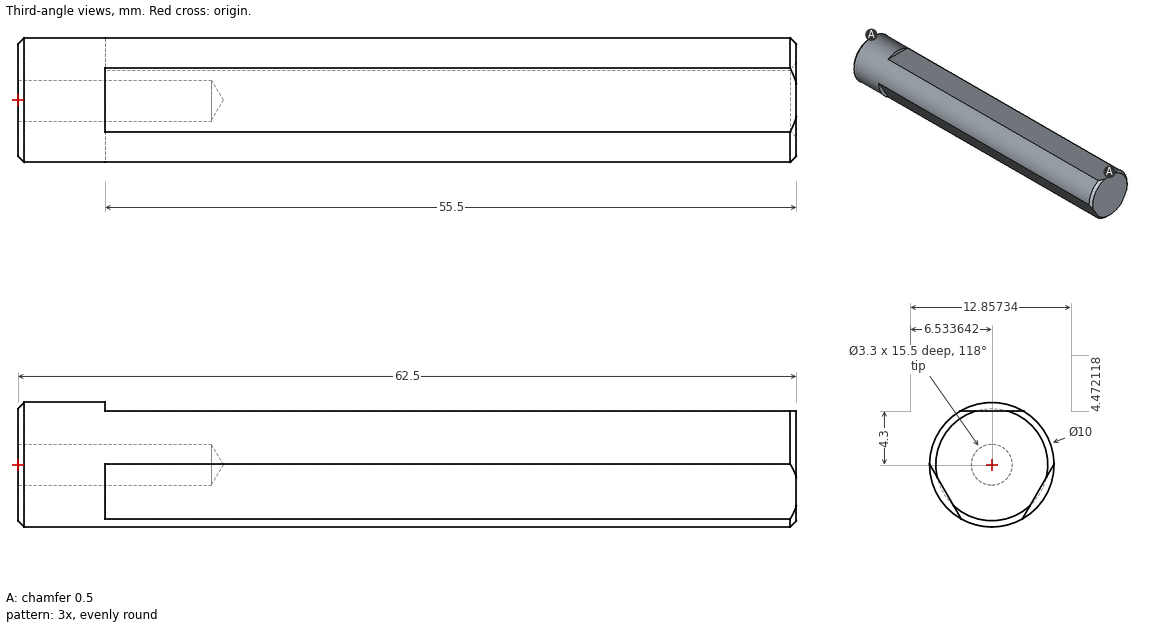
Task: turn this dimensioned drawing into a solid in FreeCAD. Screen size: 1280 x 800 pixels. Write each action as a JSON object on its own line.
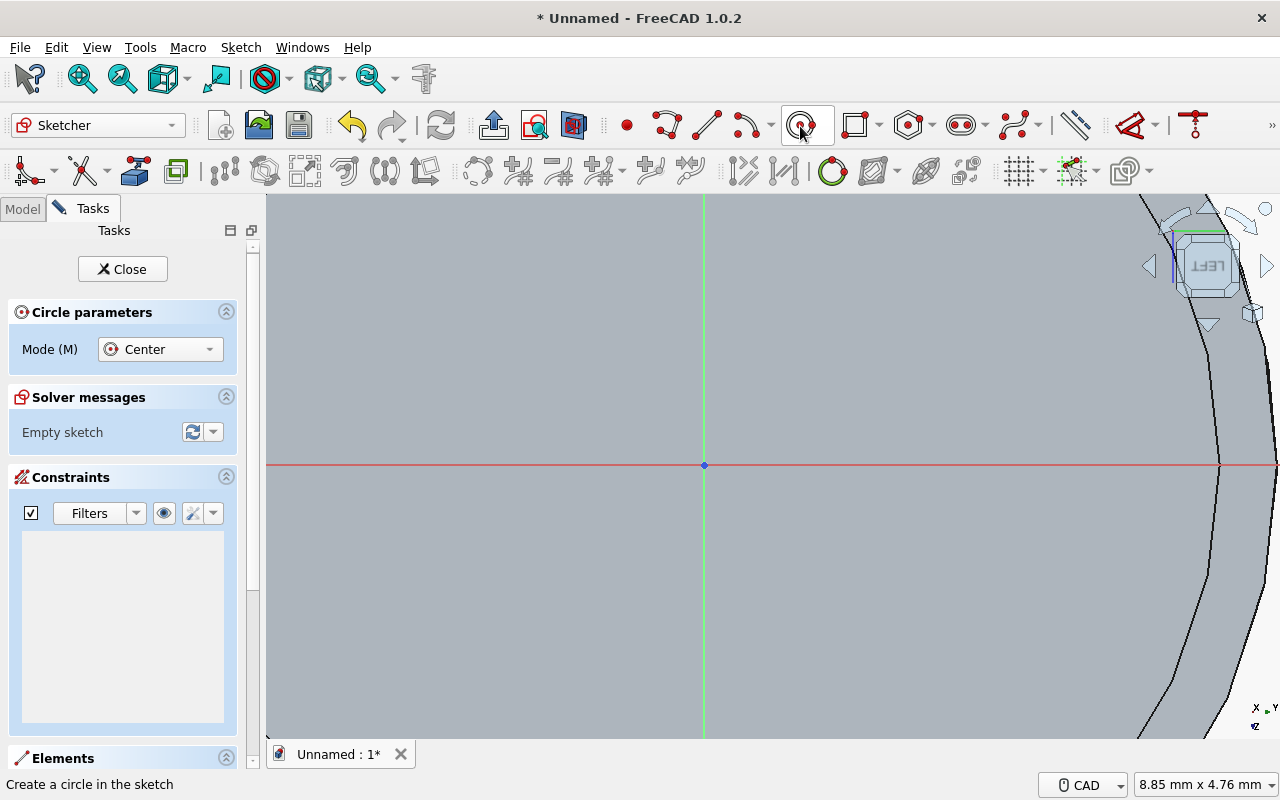
{"action": "left_click", "coordinate": [704, 465]}
{"action": "mouse_move", "coordinate": [838, 331]}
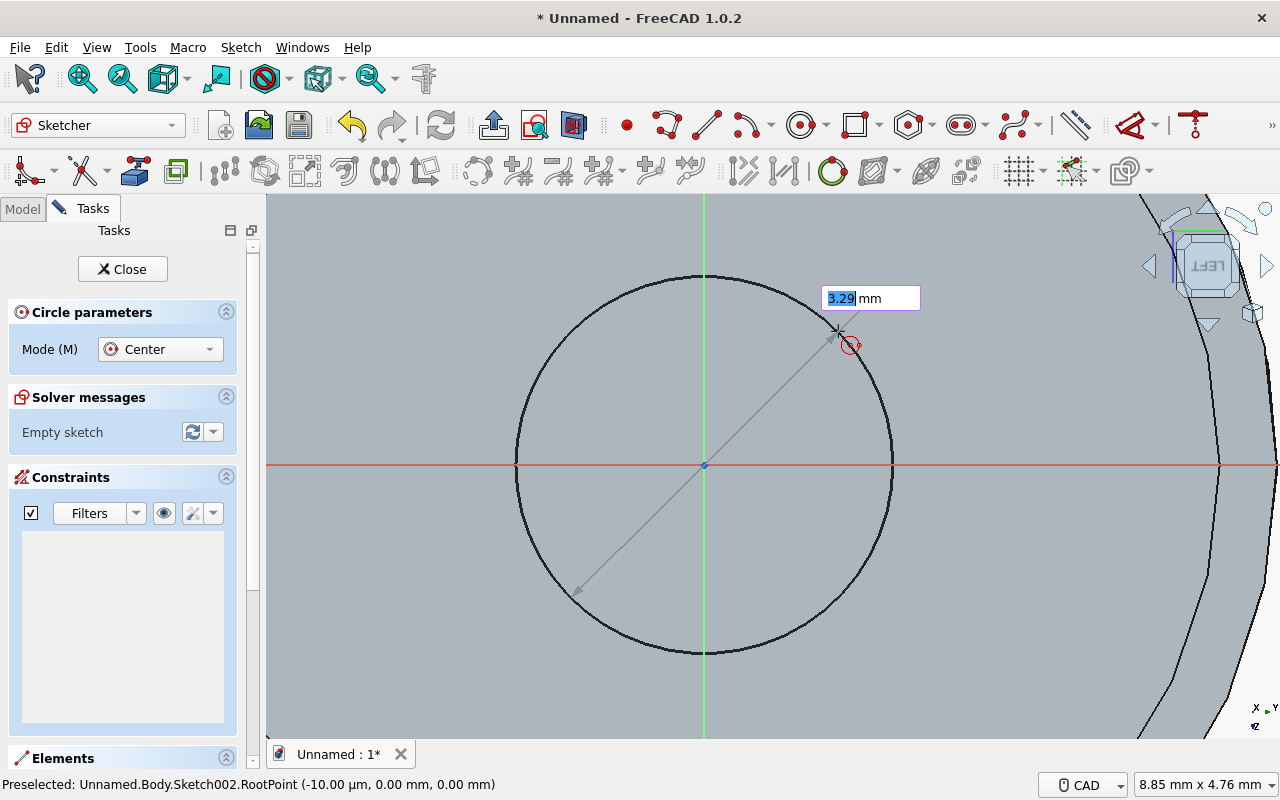
{"action": "type", "text": "3.3"}
{"action": "key", "text": "Return"}
{"action": "key", "text": "Escape"}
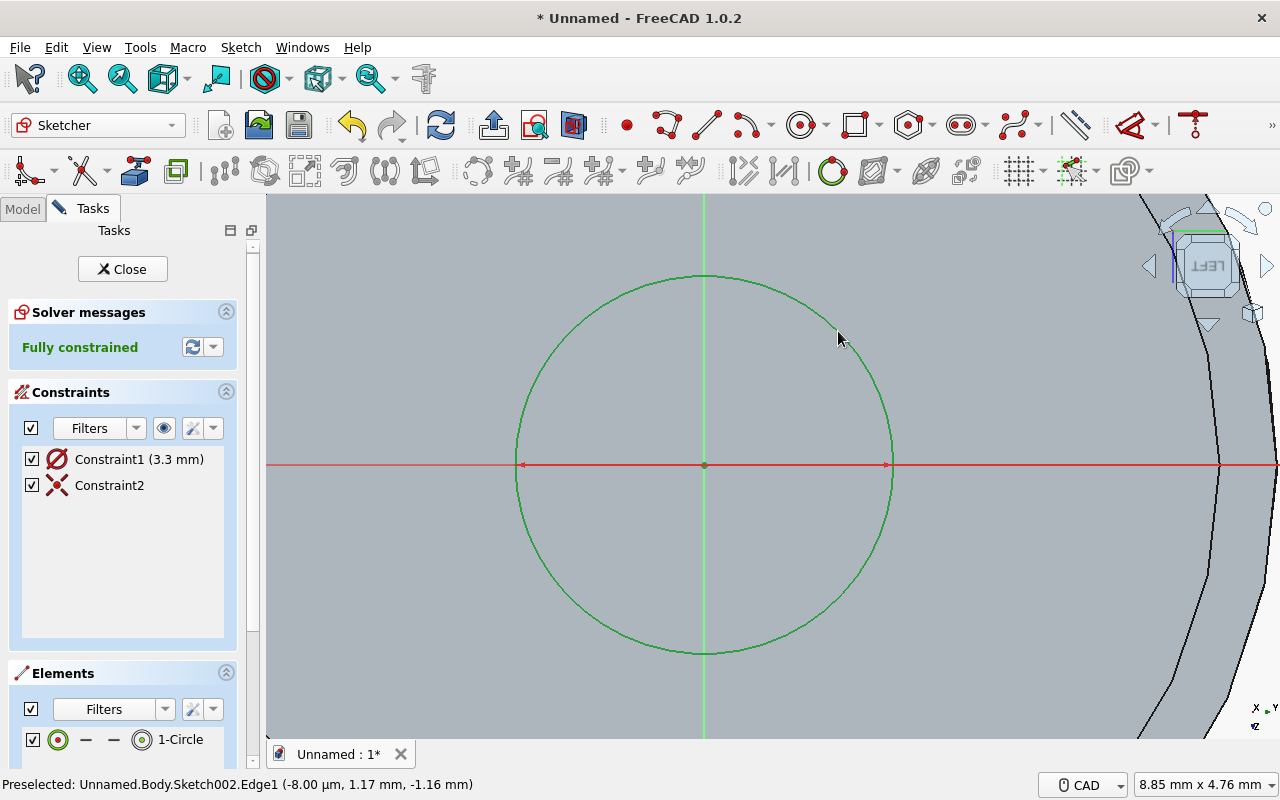
{"action": "left_click", "coordinate": [123, 269]}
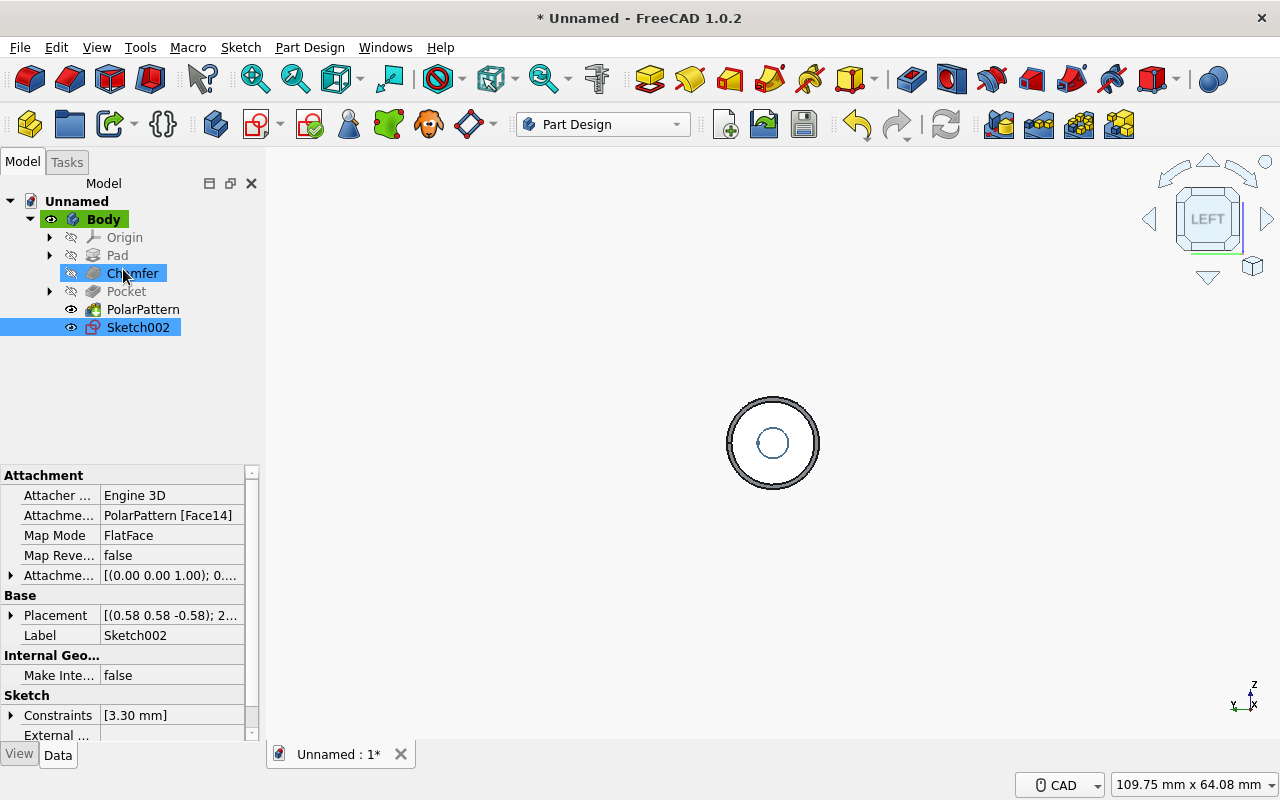
{"action": "left_click", "coordinate": [952, 80]}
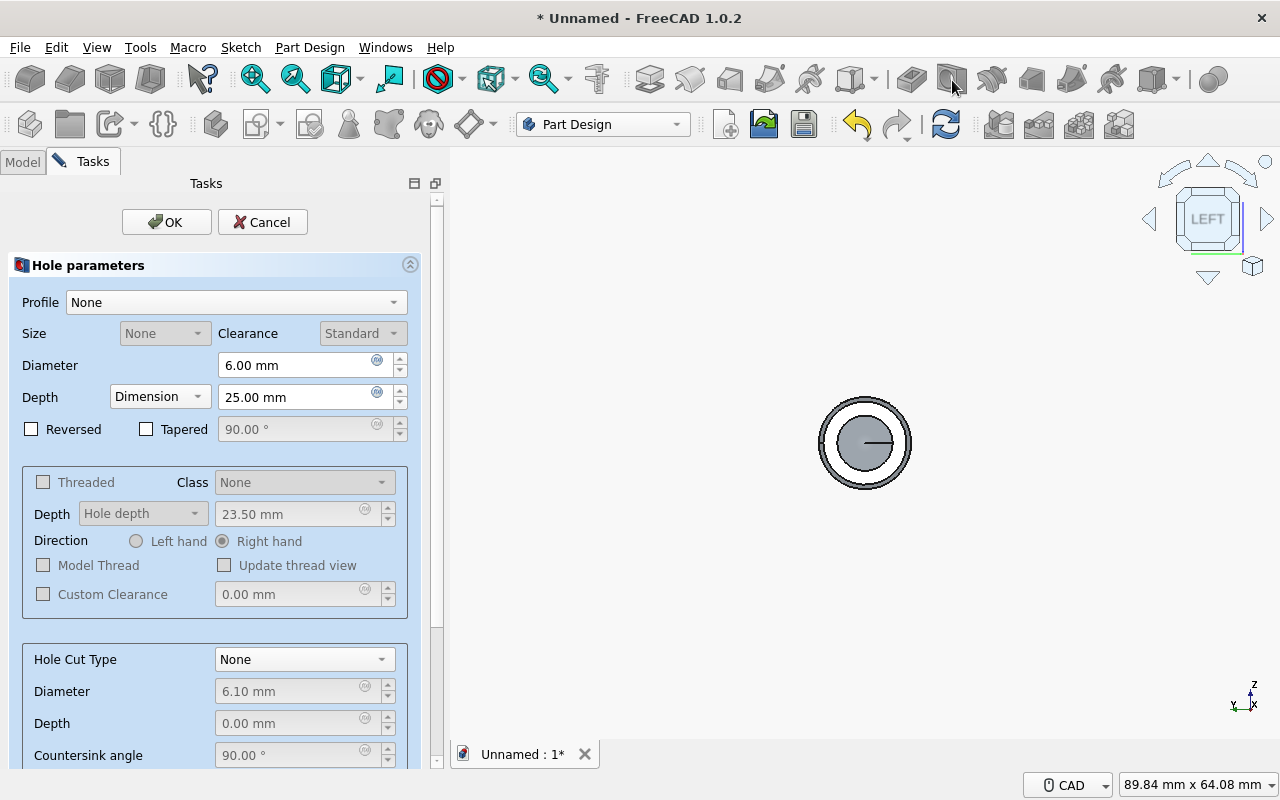
{"action": "triple_click", "coordinate": [305, 365]}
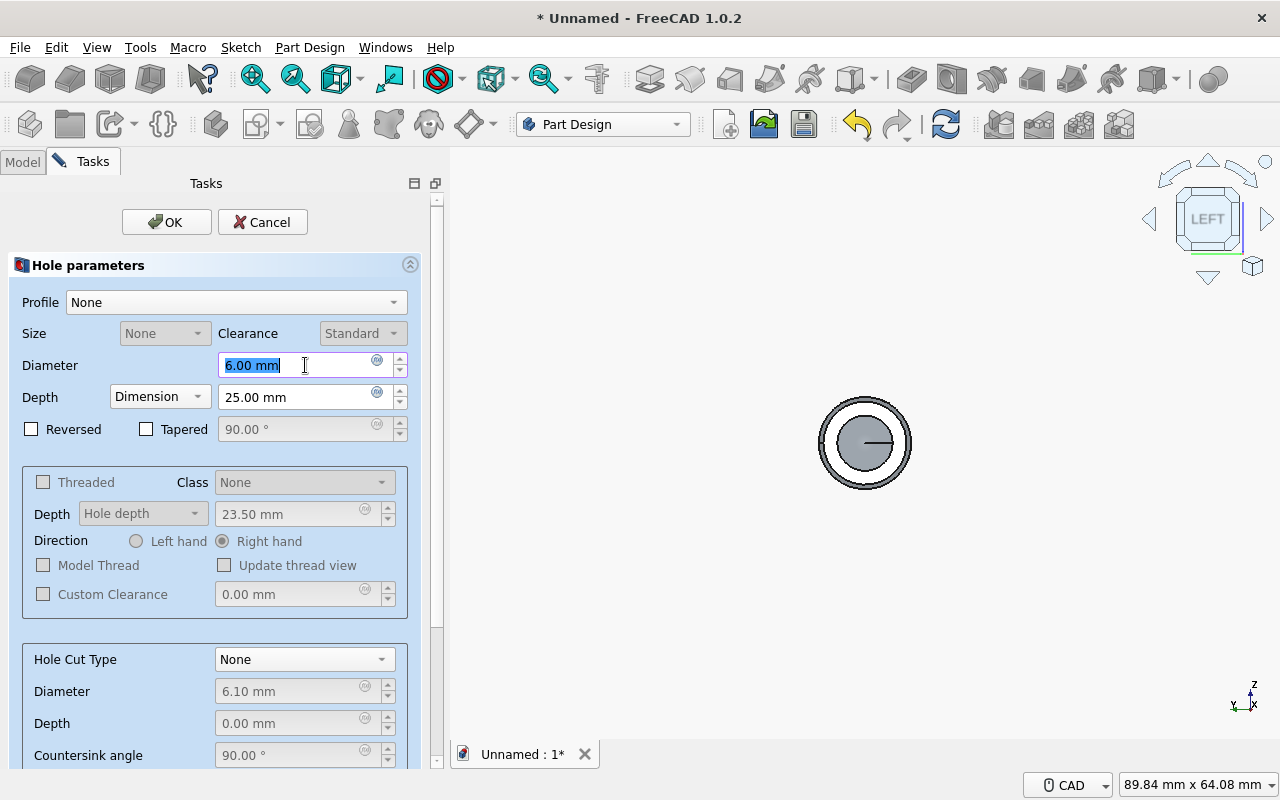
{"action": "type", "text": "3.3"}
{"action": "key", "text": "Tab"}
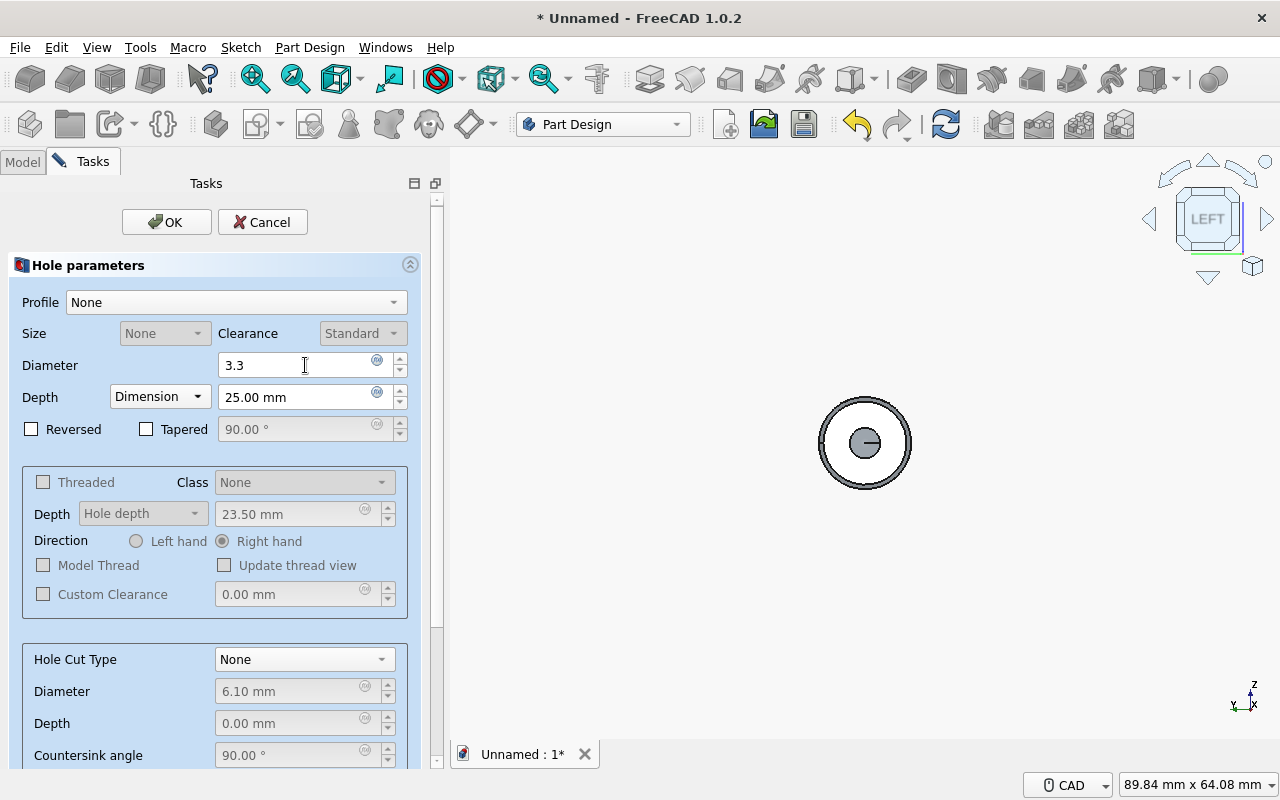
{"action": "triple_click", "coordinate": [305, 397]}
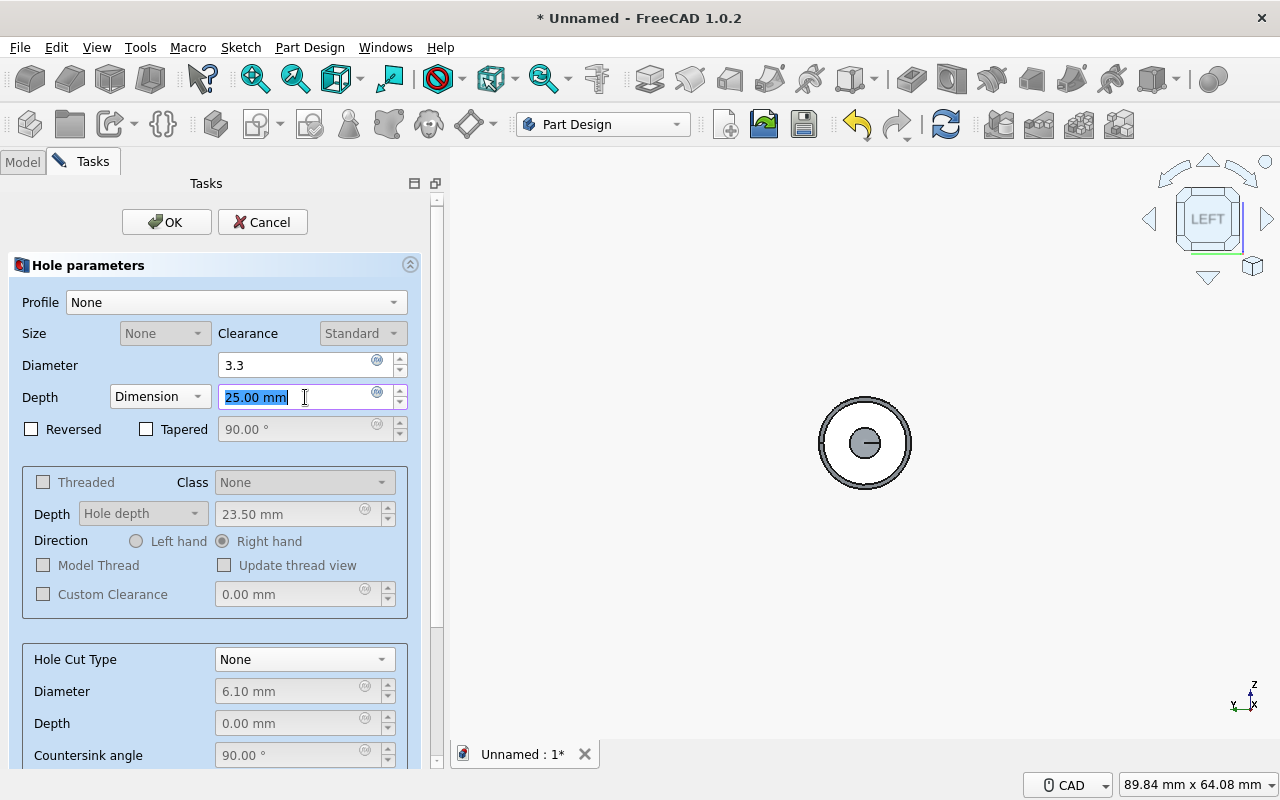
{"action": "type", "text": "15.5"}
{"action": "key", "text": "Tab"}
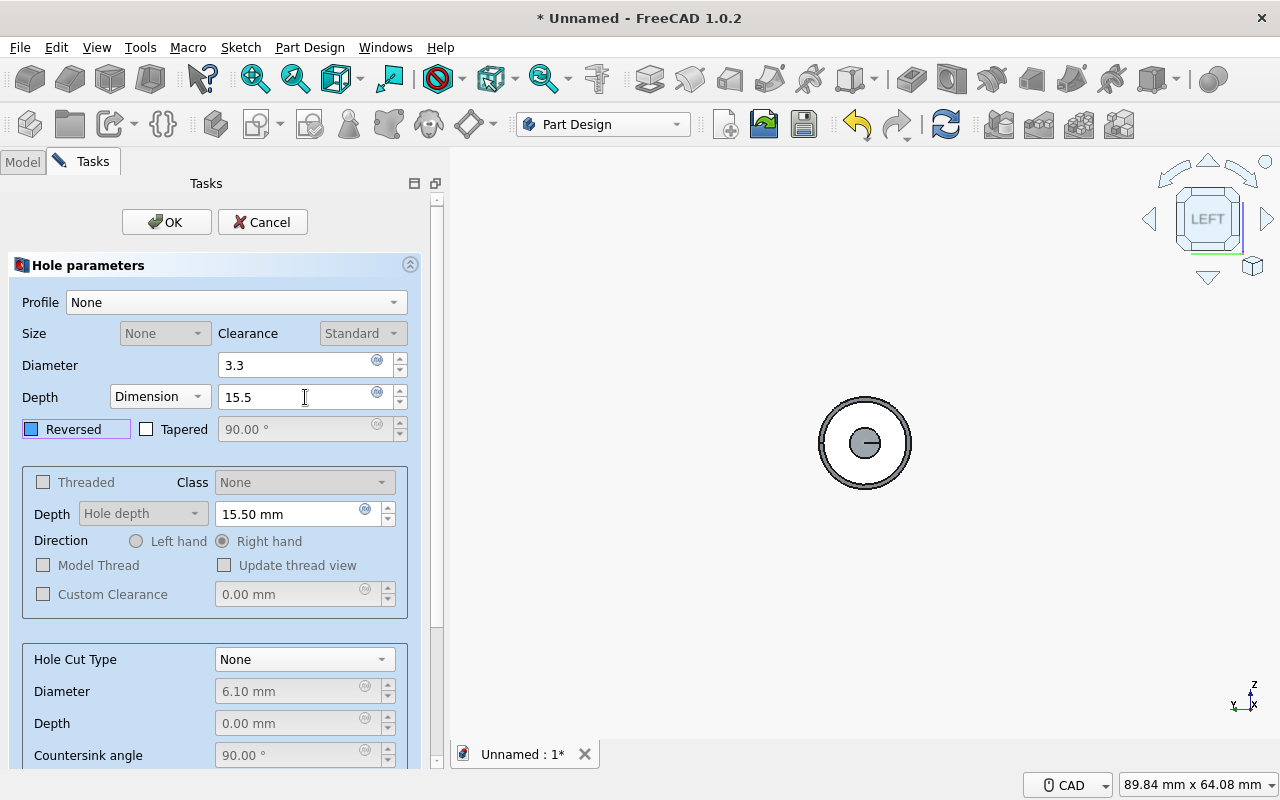
{"action": "left_click", "coordinate": [167, 222]}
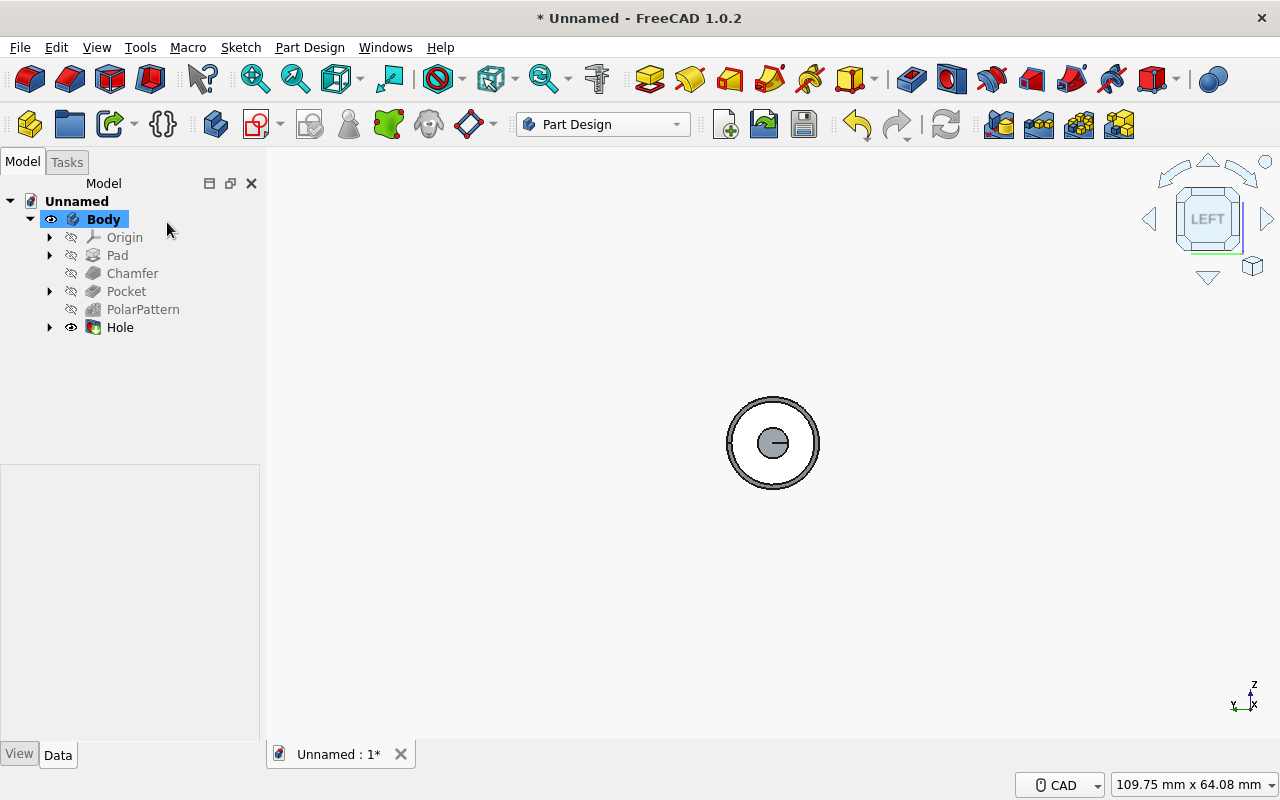
{"action": "key", "text": "0"}